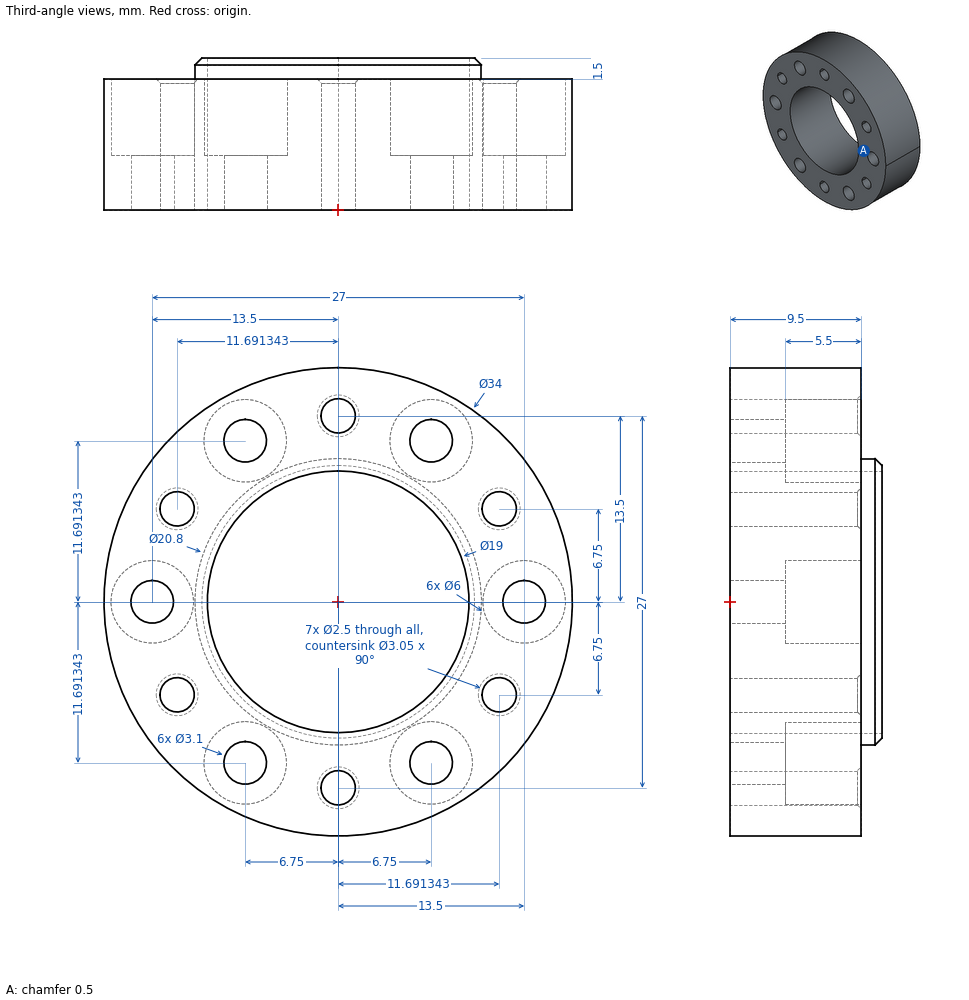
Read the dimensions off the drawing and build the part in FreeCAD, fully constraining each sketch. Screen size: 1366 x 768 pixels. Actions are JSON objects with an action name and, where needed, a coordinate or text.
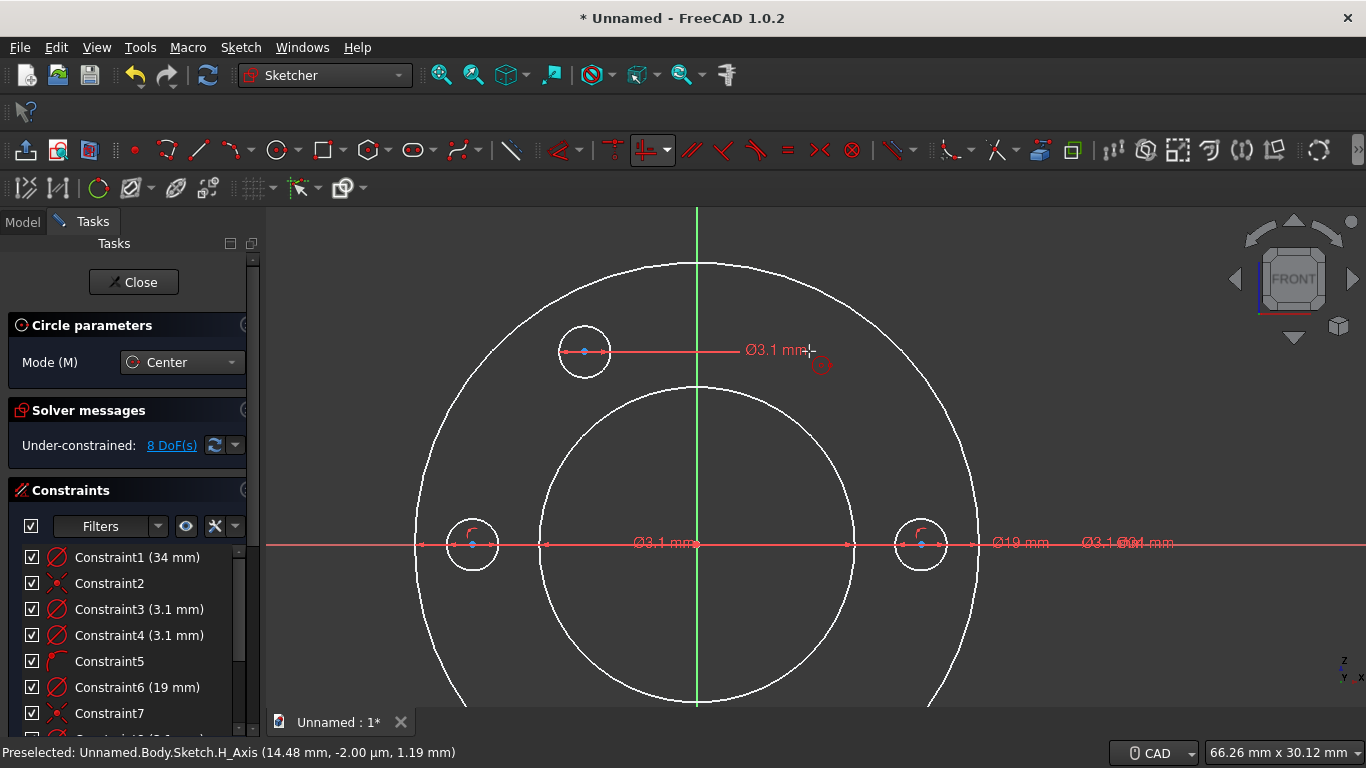
{"action": "left_click", "coordinate": [809, 351]}
{"action": "mouse_move", "coordinate": [827, 333]}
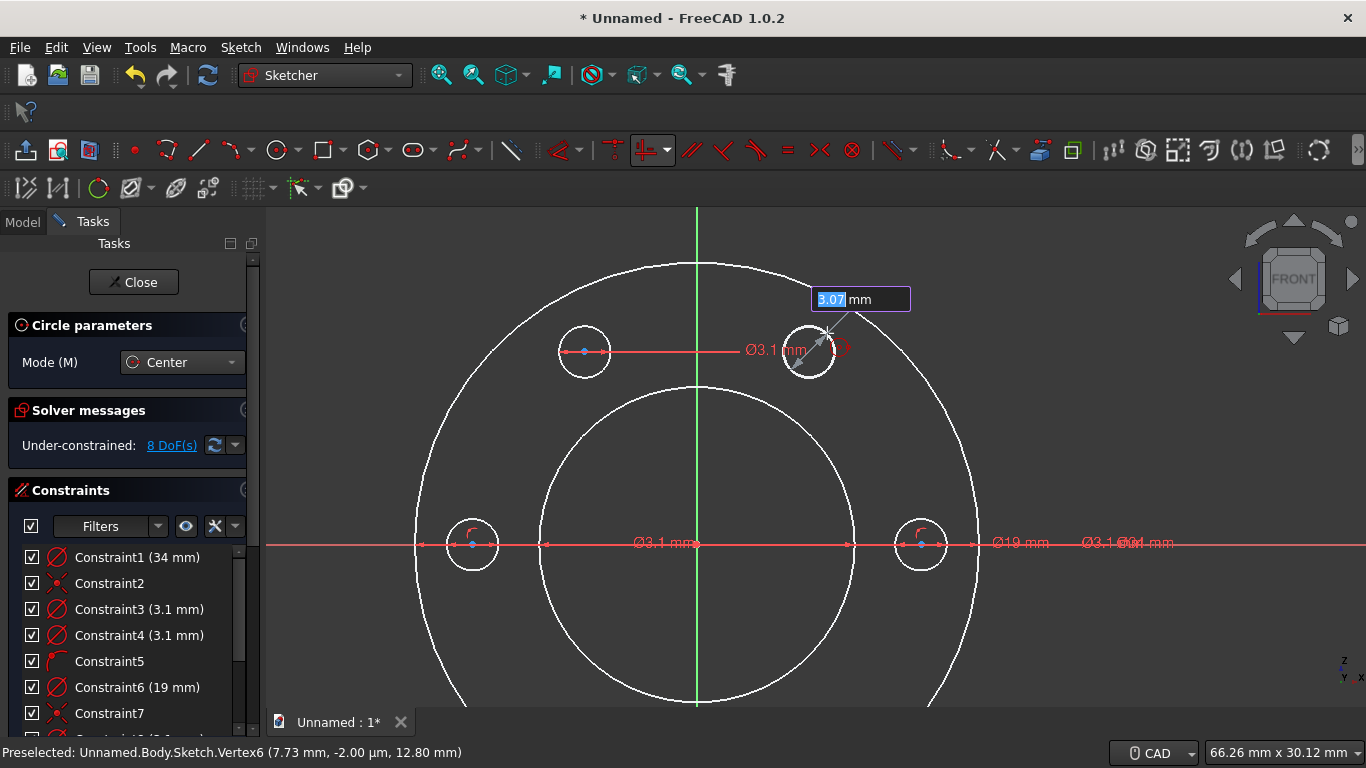
{"action": "type", "text": "3.1"}
{"action": "key", "text": "Return"}
{"action": "key", "text": "Escape"}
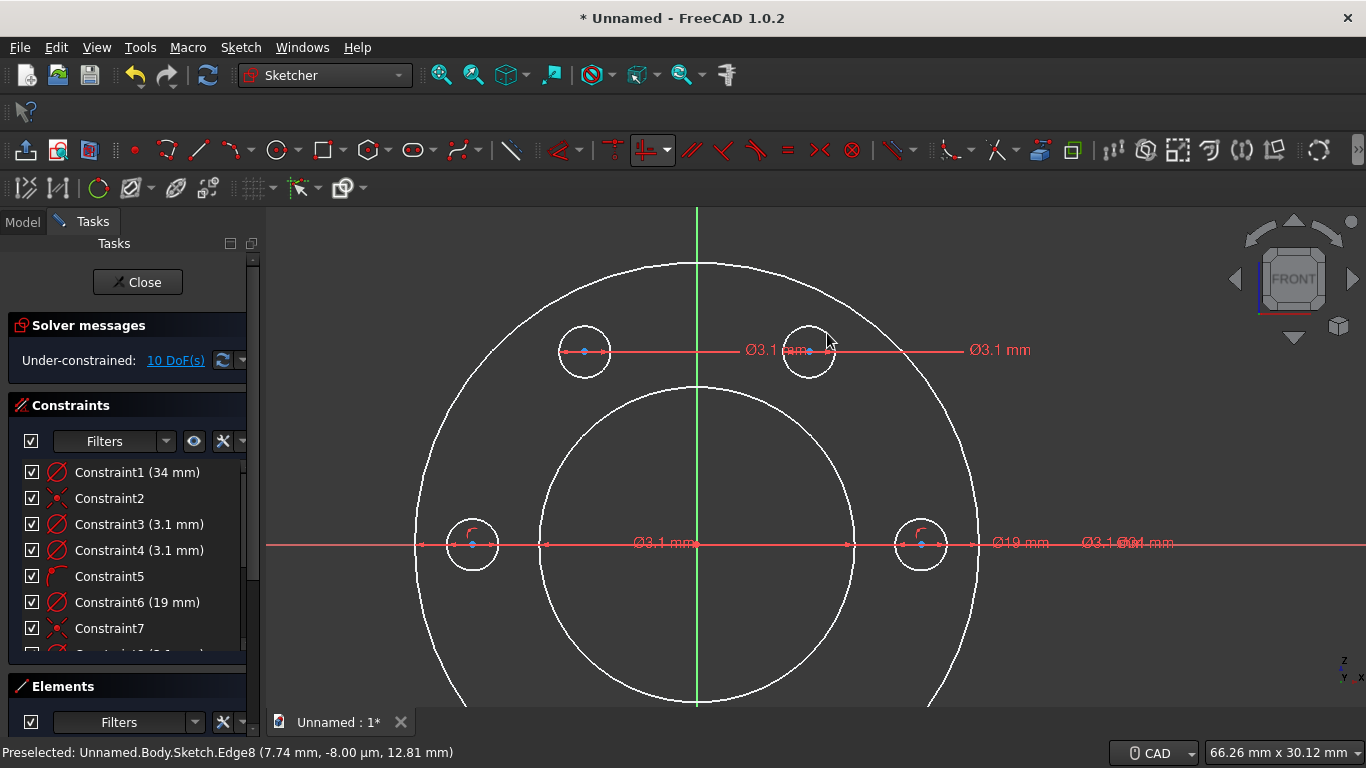
{"action": "scroll", "coordinate": [809, 350], "scroll_direction": "down", "scroll_amount": 3}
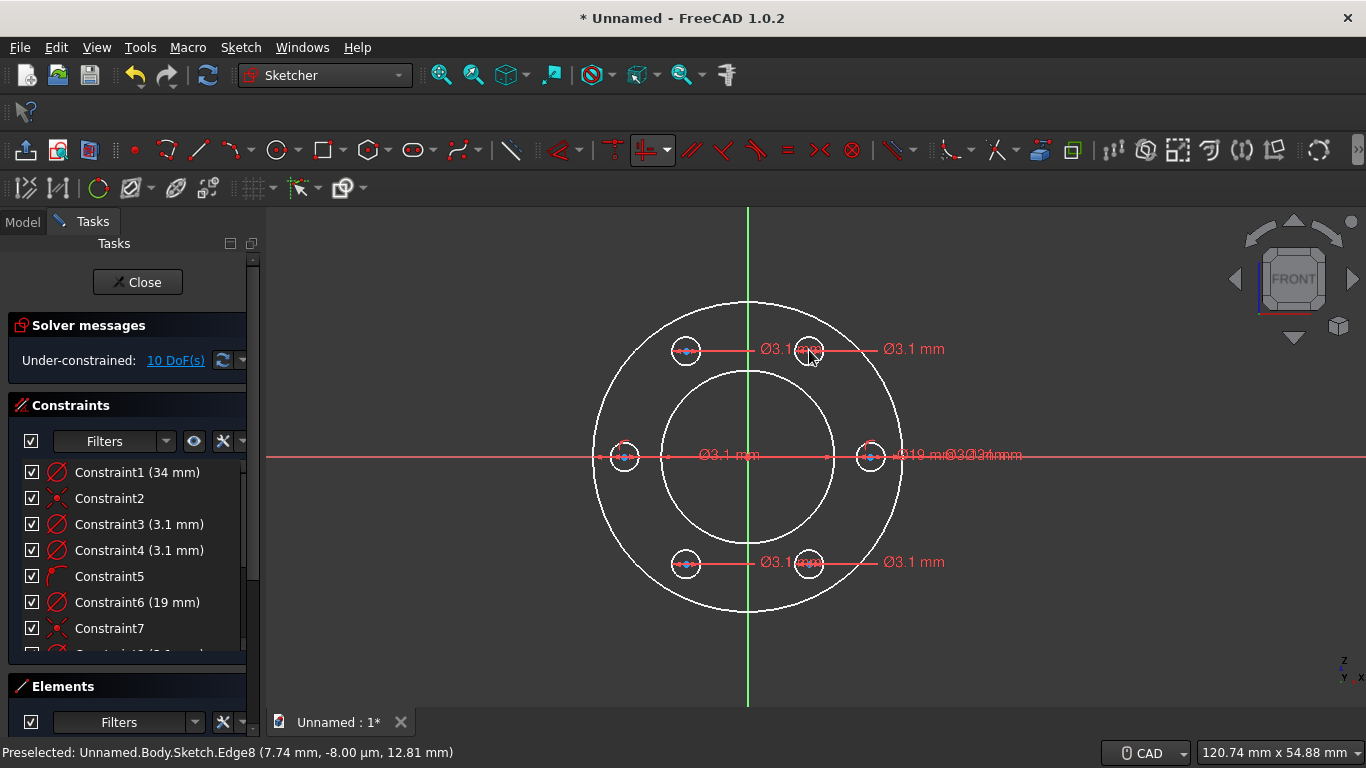
{"action": "left_click", "coordinate": [686, 564]}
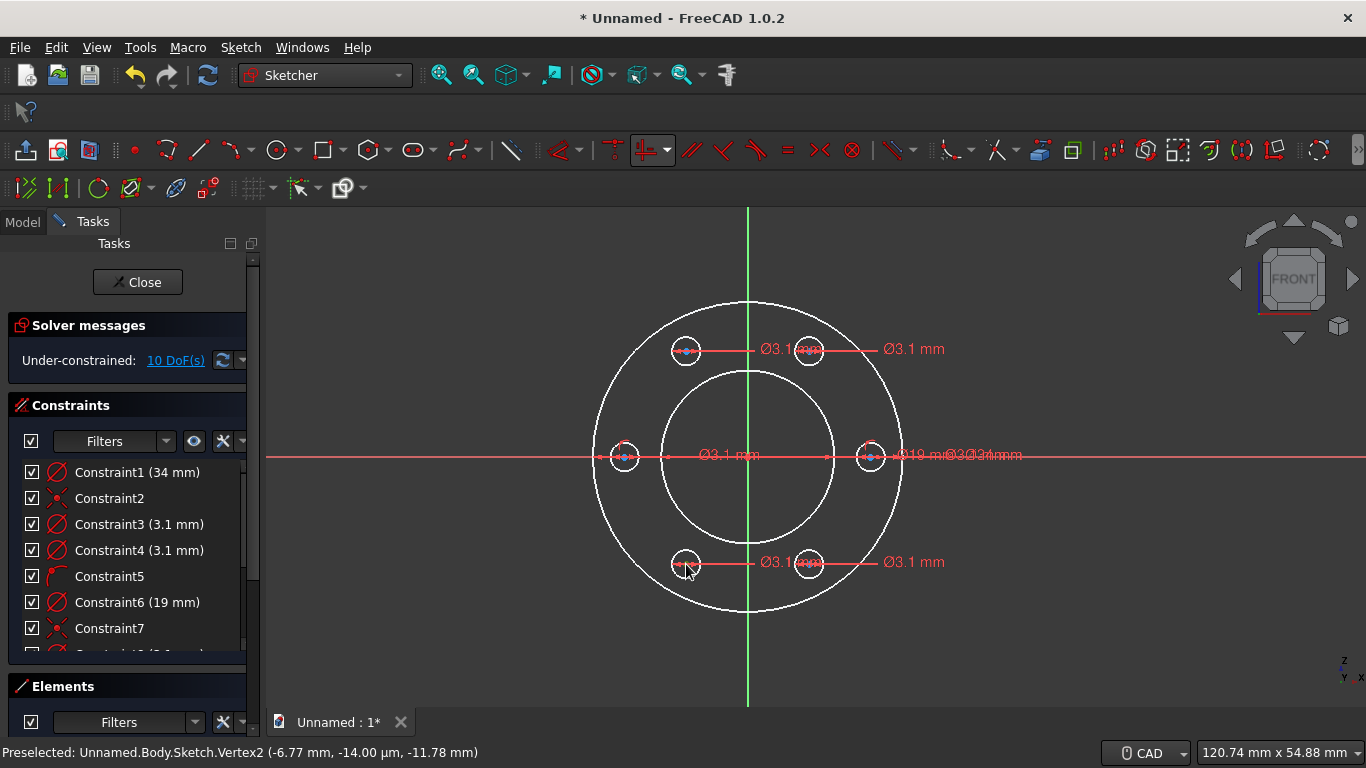
{"action": "left_click", "coordinate": [686, 351]}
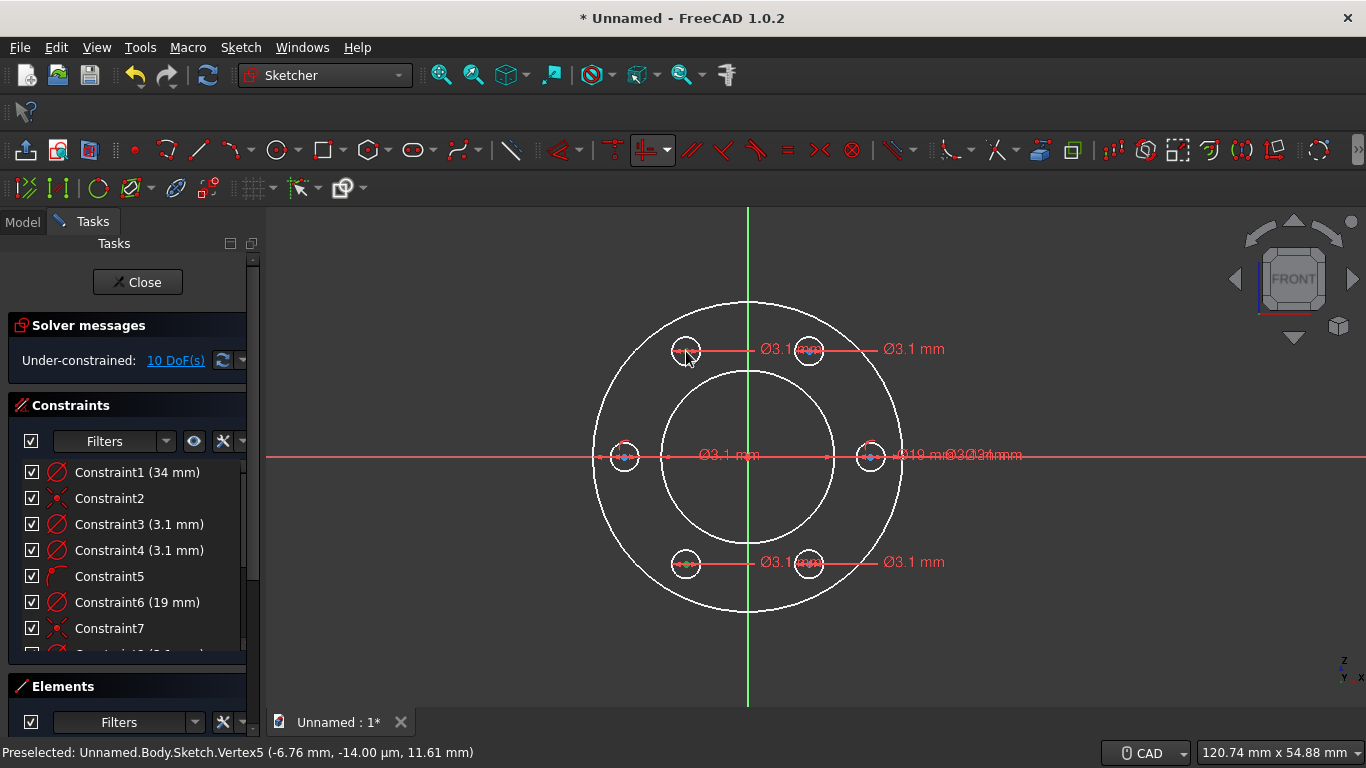
{"action": "left_click", "coordinate": [670, 150]}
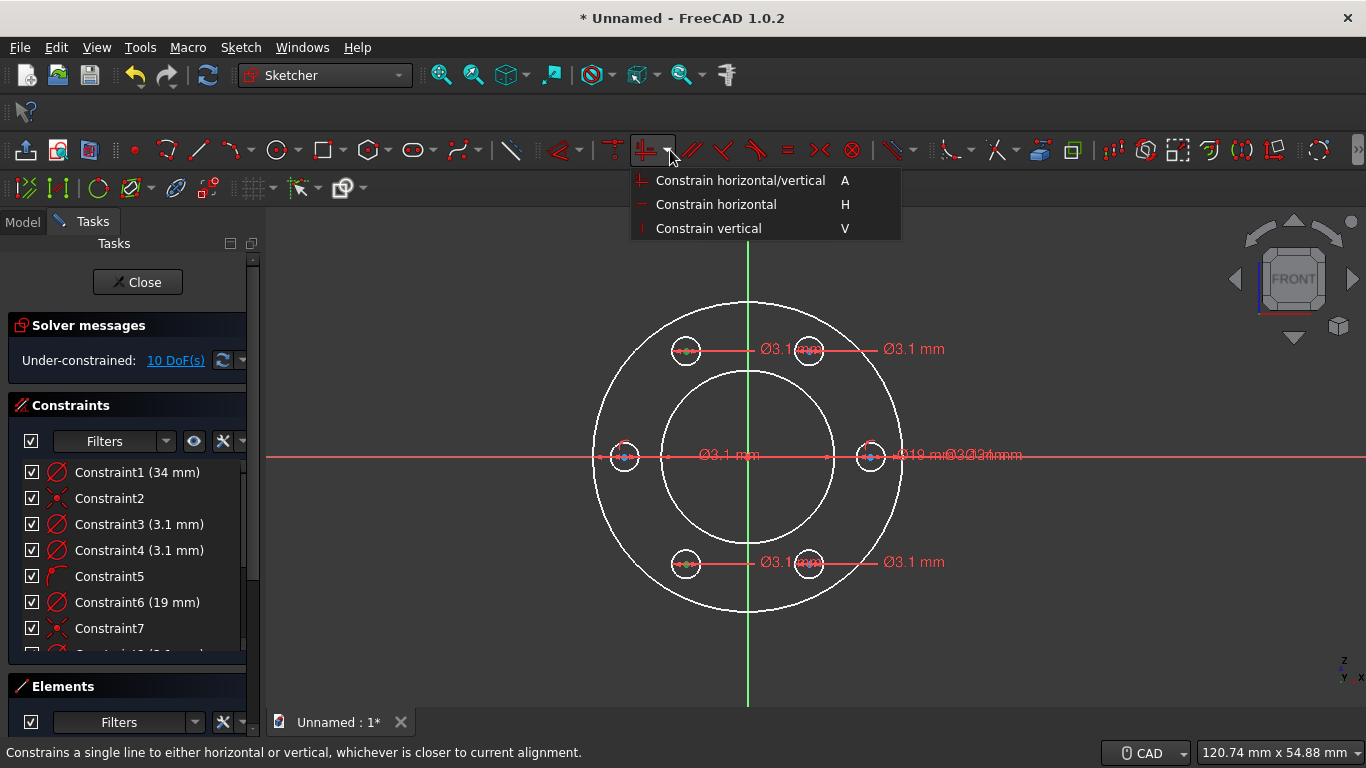
{"action": "left_click", "coordinate": [766, 228]}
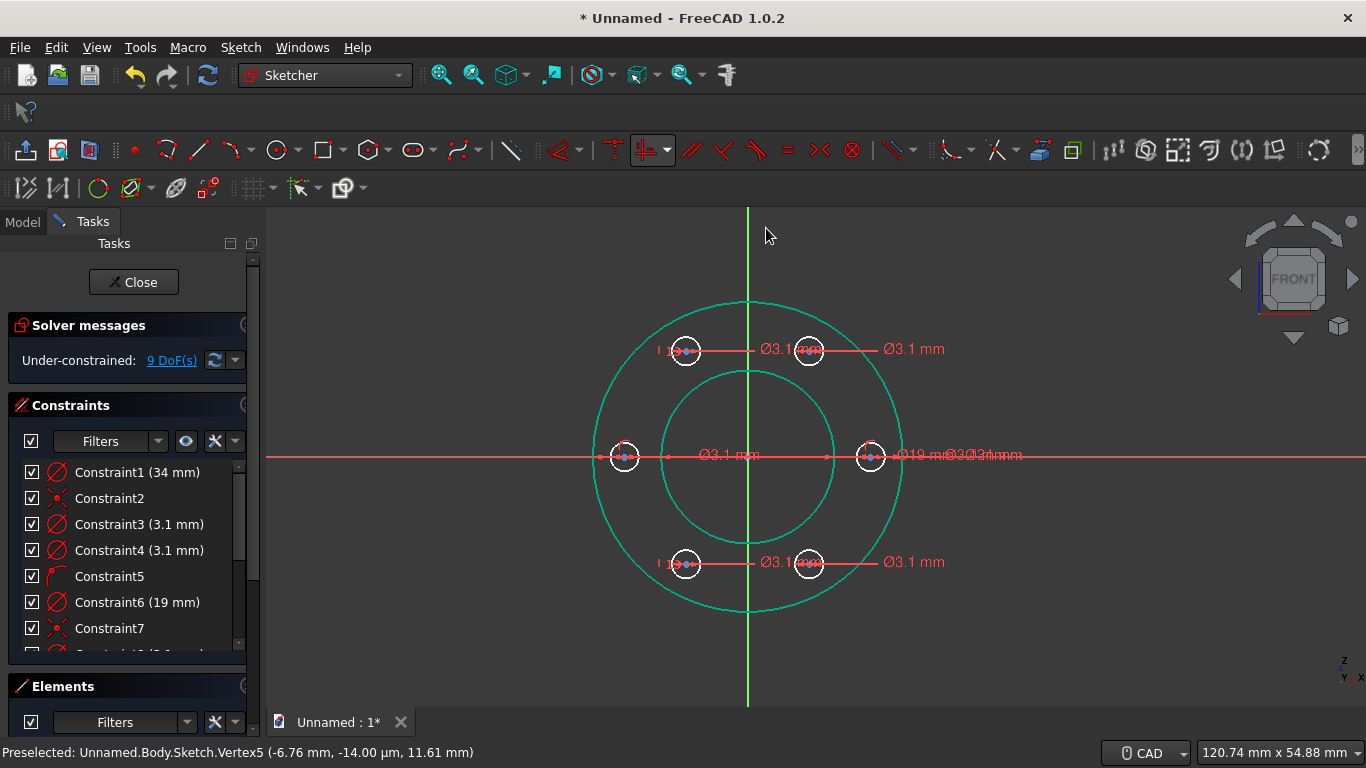
{"action": "left_click", "coordinate": [686, 564]}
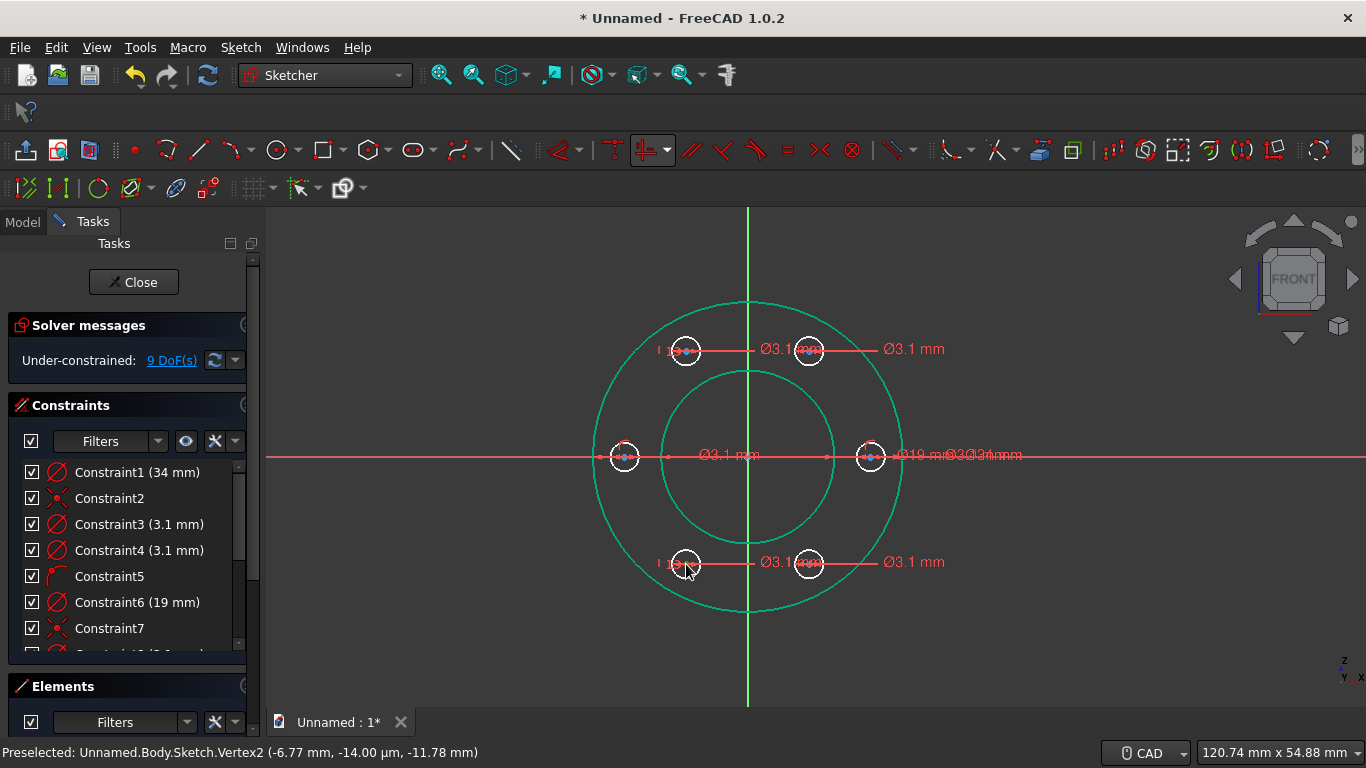
{"action": "left_click", "coordinate": [809, 564]}